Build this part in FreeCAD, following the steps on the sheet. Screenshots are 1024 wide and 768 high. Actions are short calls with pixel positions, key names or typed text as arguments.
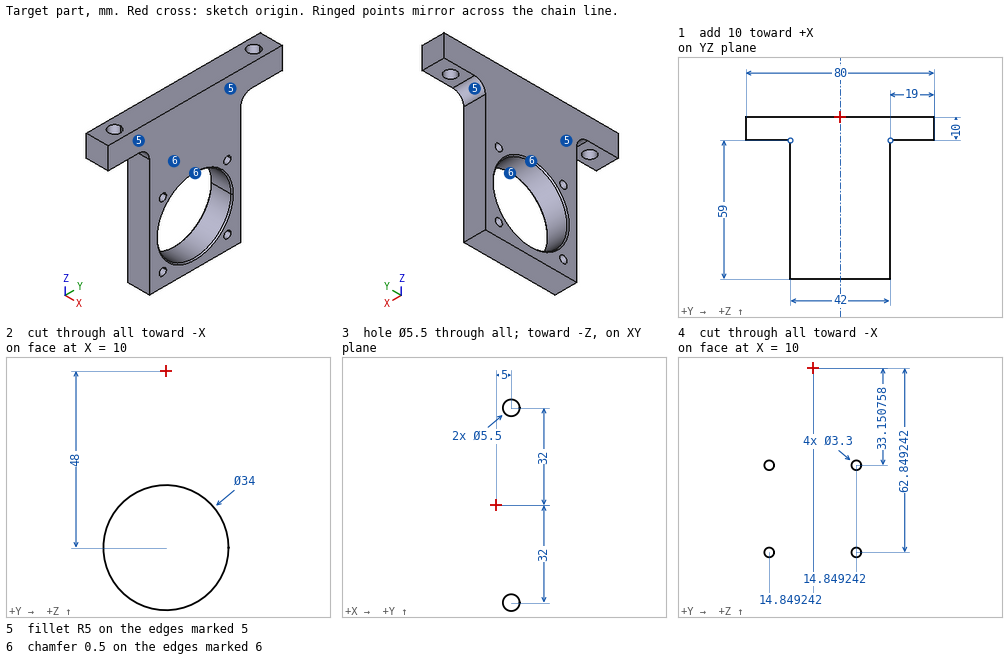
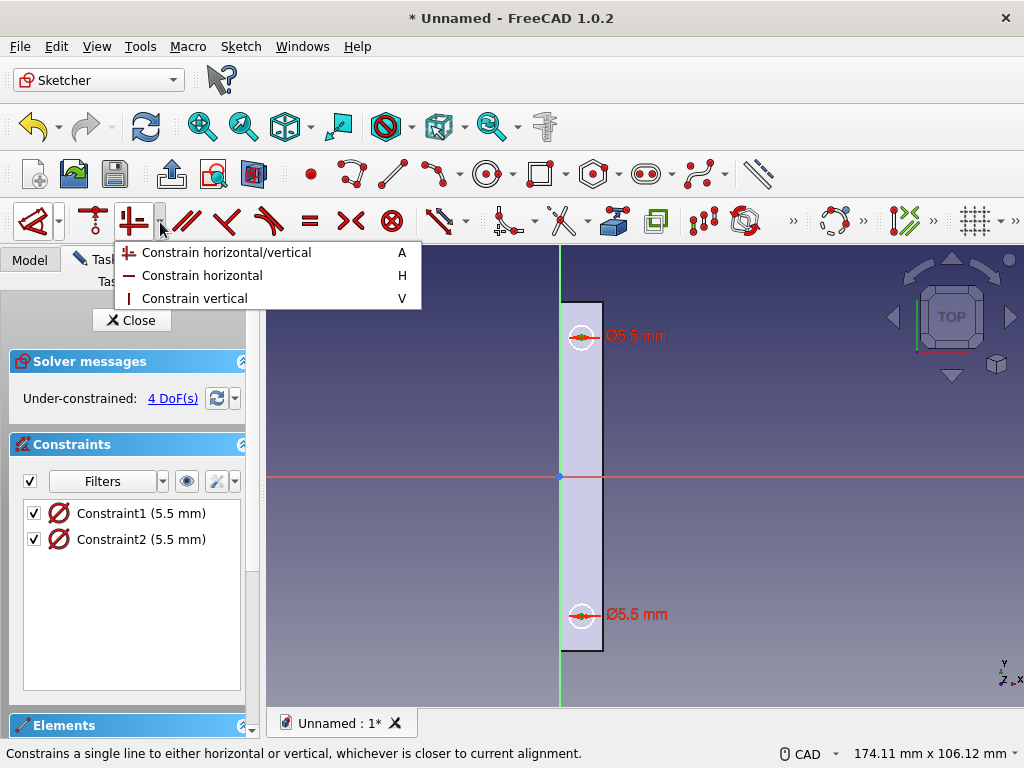
click(268, 298)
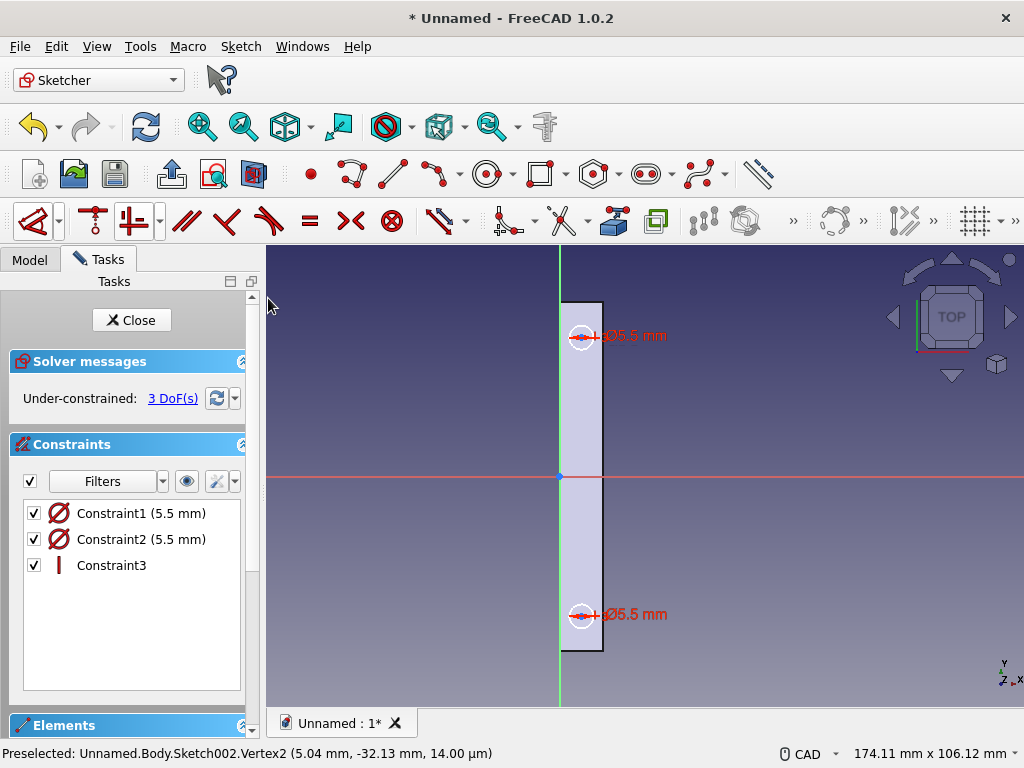
scroll(581, 338, up, 4)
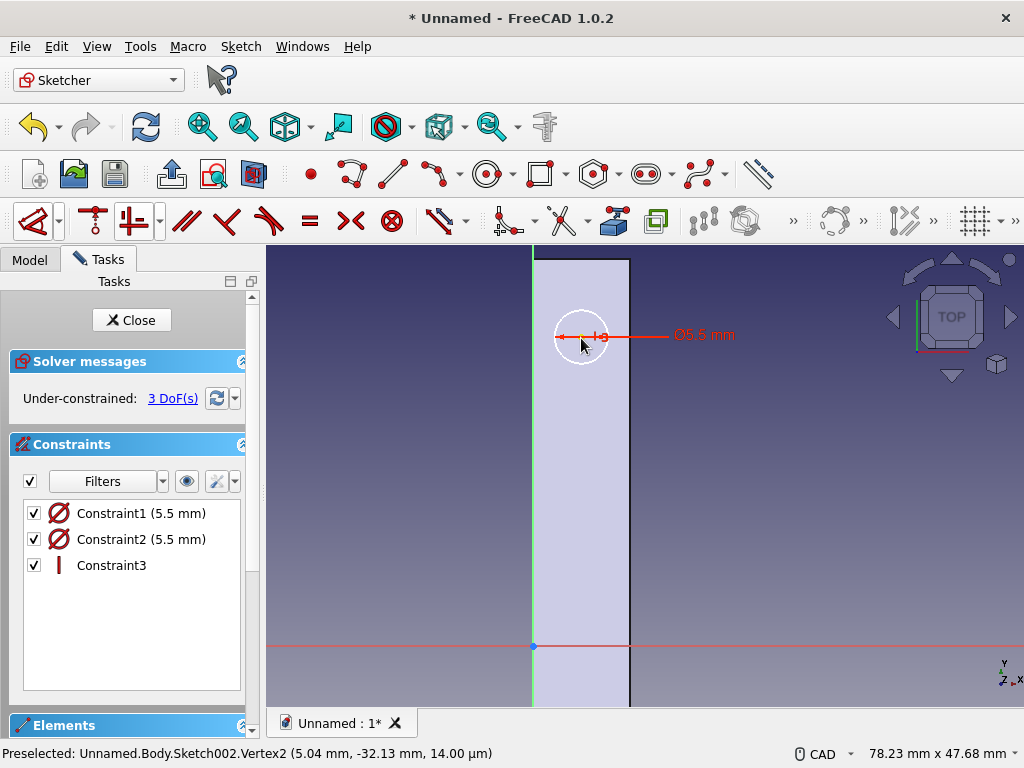
click(581, 337)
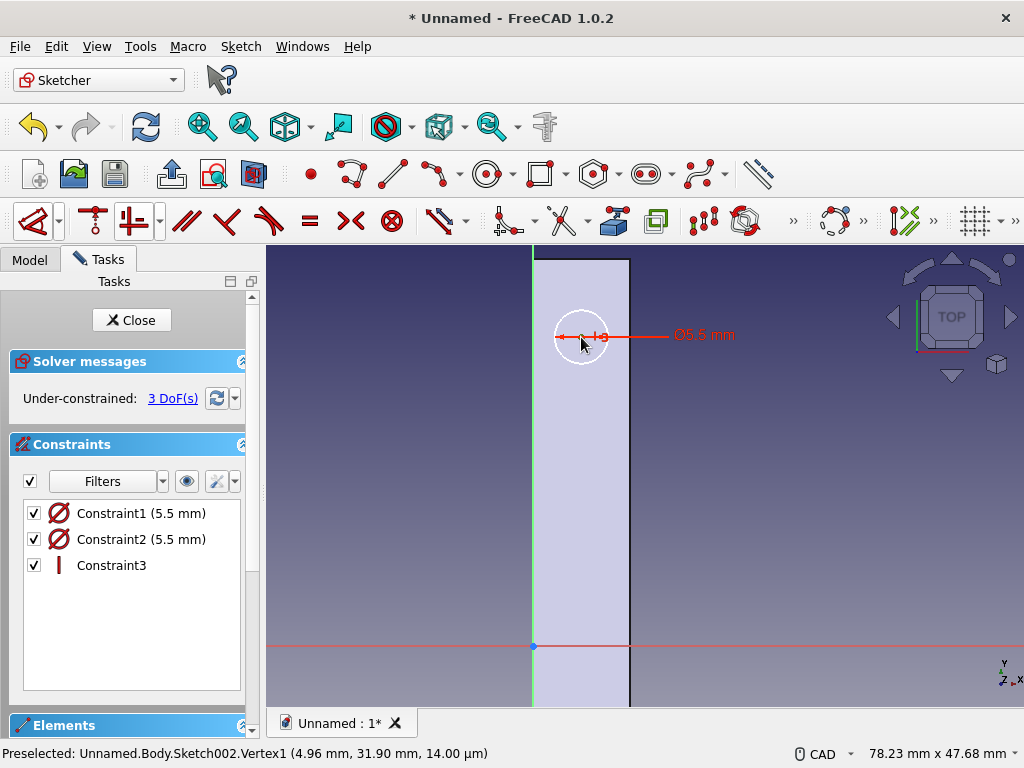
key(l)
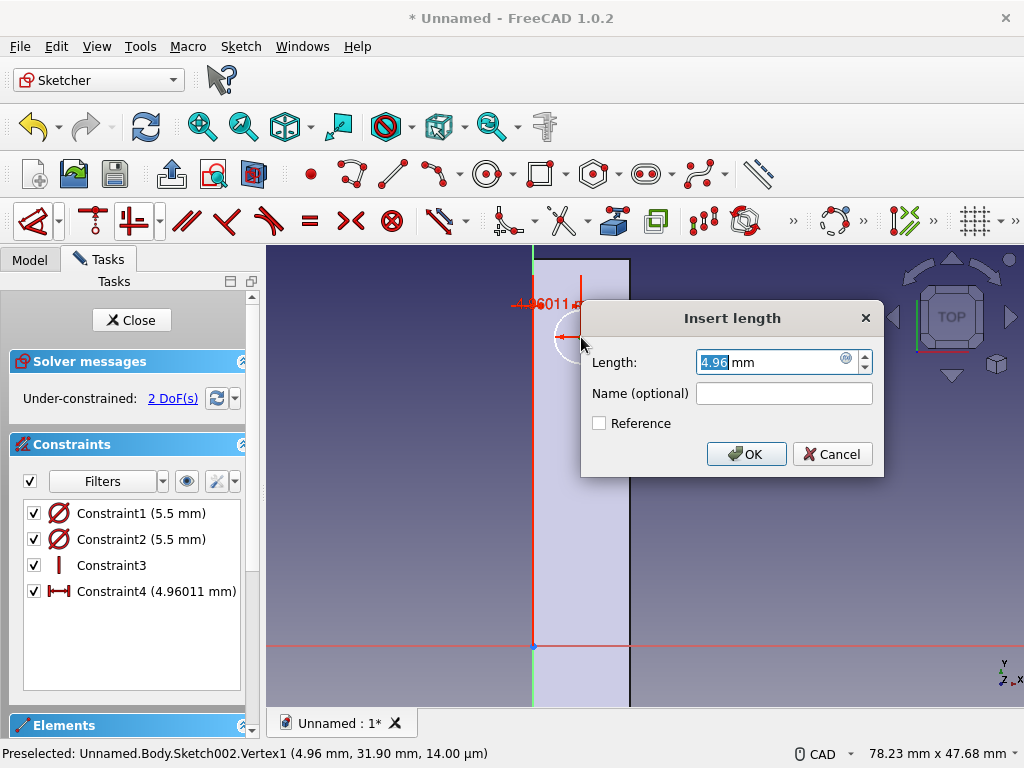
text(5)
key(Return)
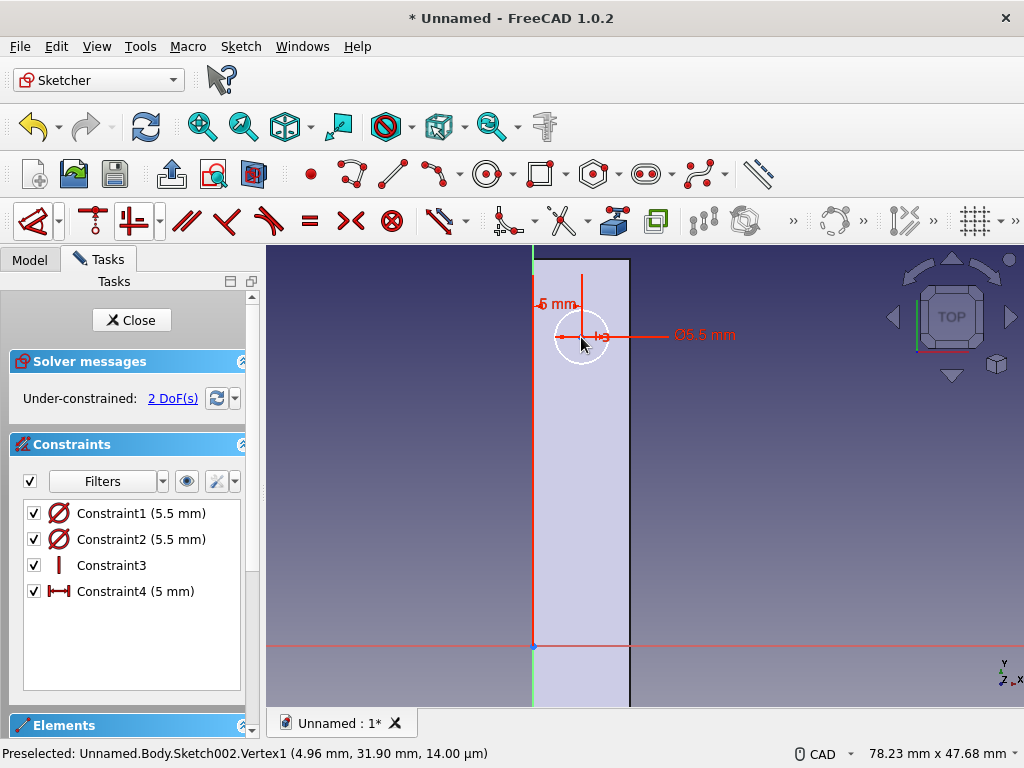
click(582, 337)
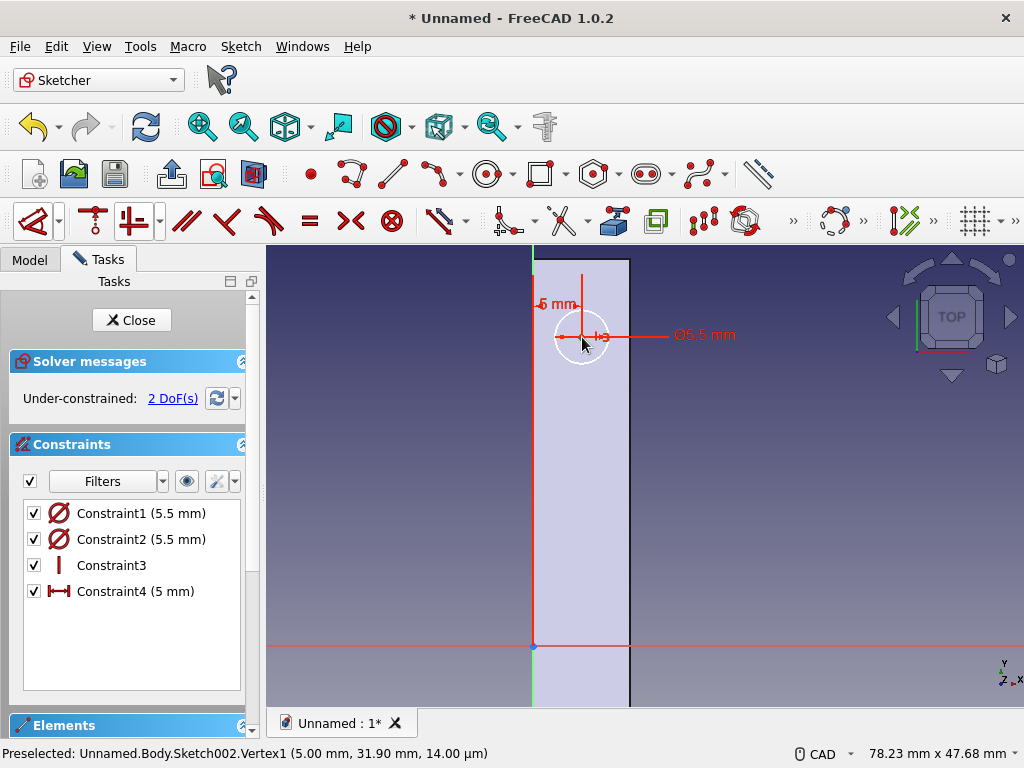
click(58, 222)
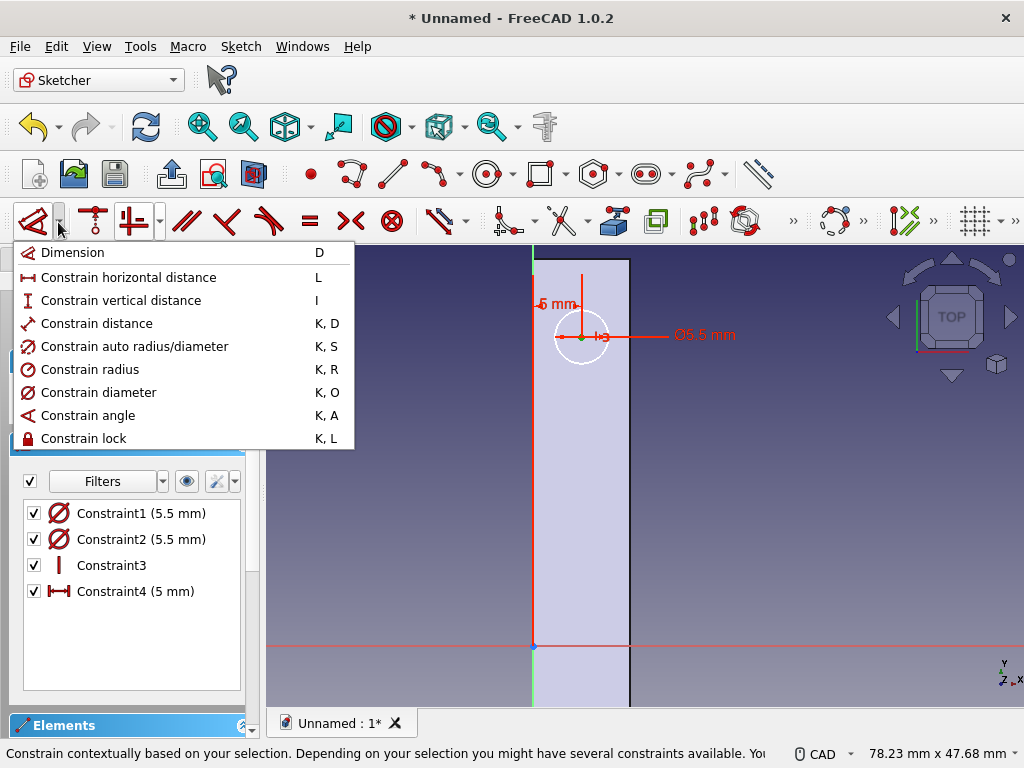
click(184, 300)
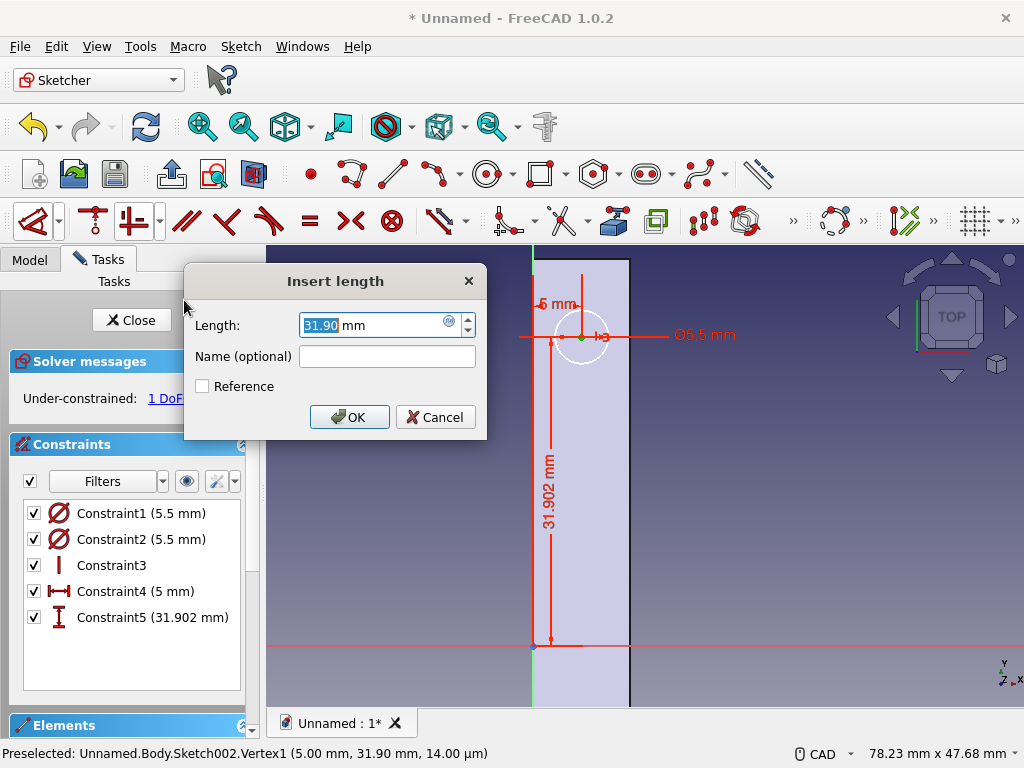
text(32)
key(Return)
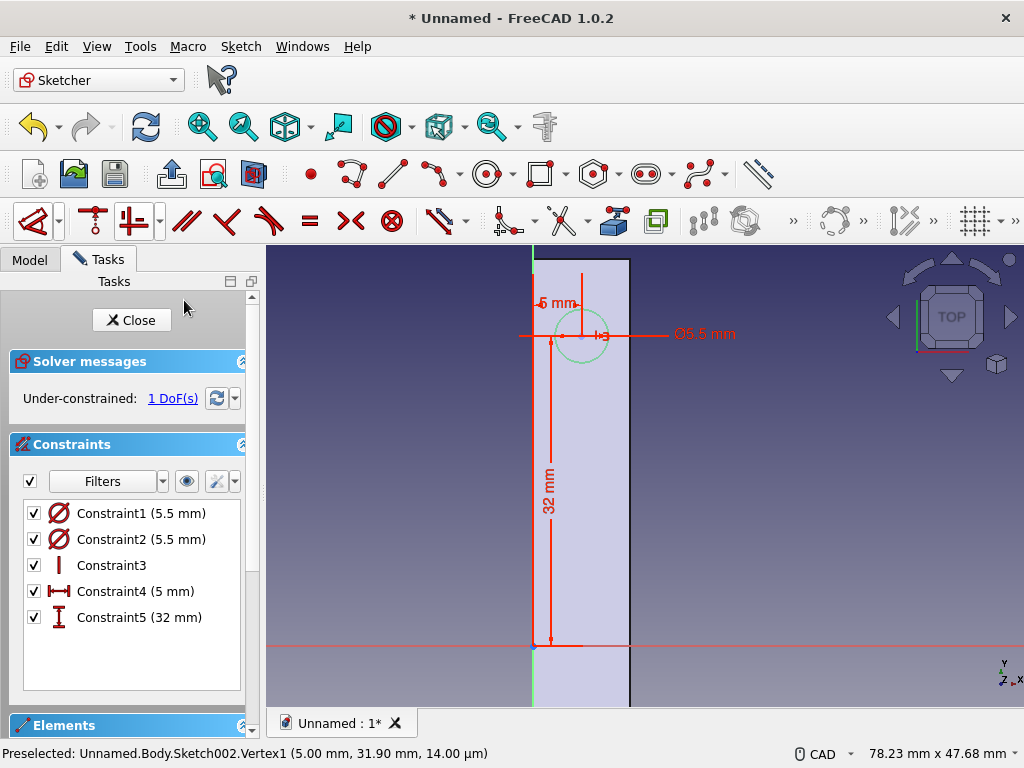
scroll(581, 337, down, 4)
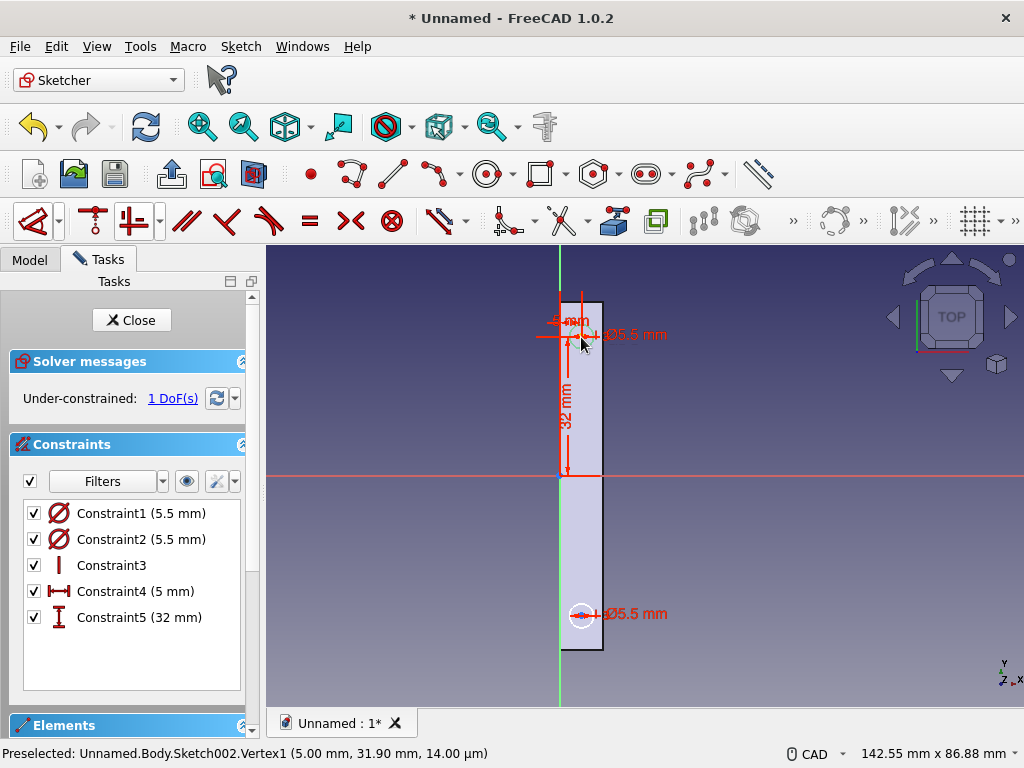
click(582, 616)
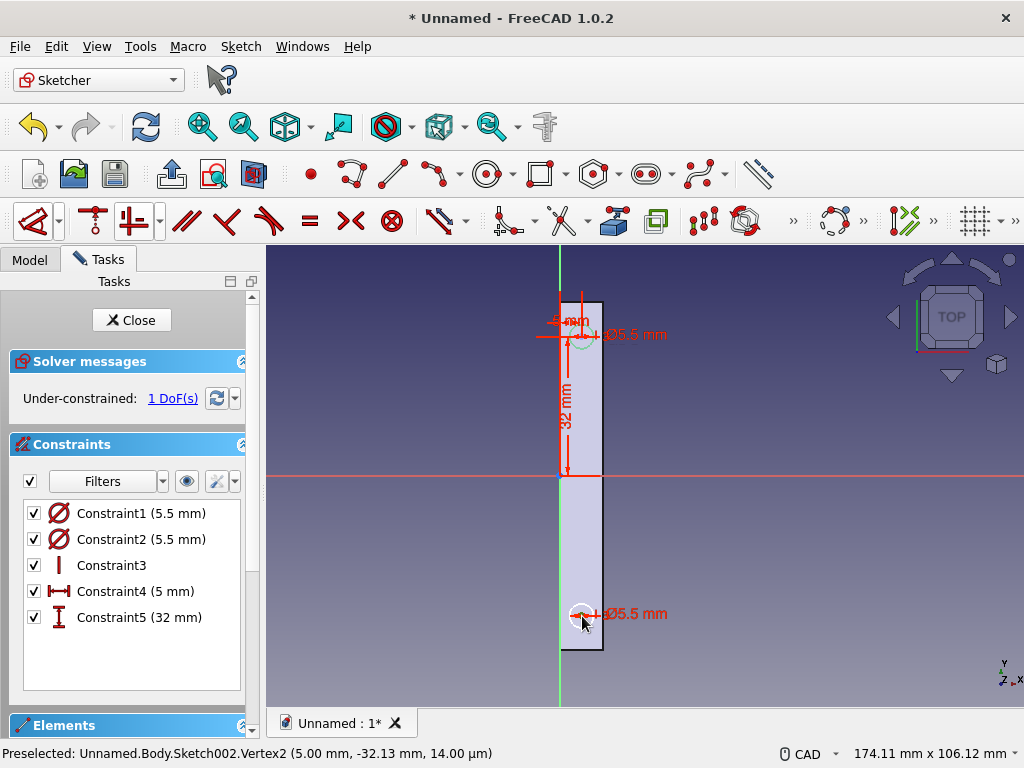
click(58, 222)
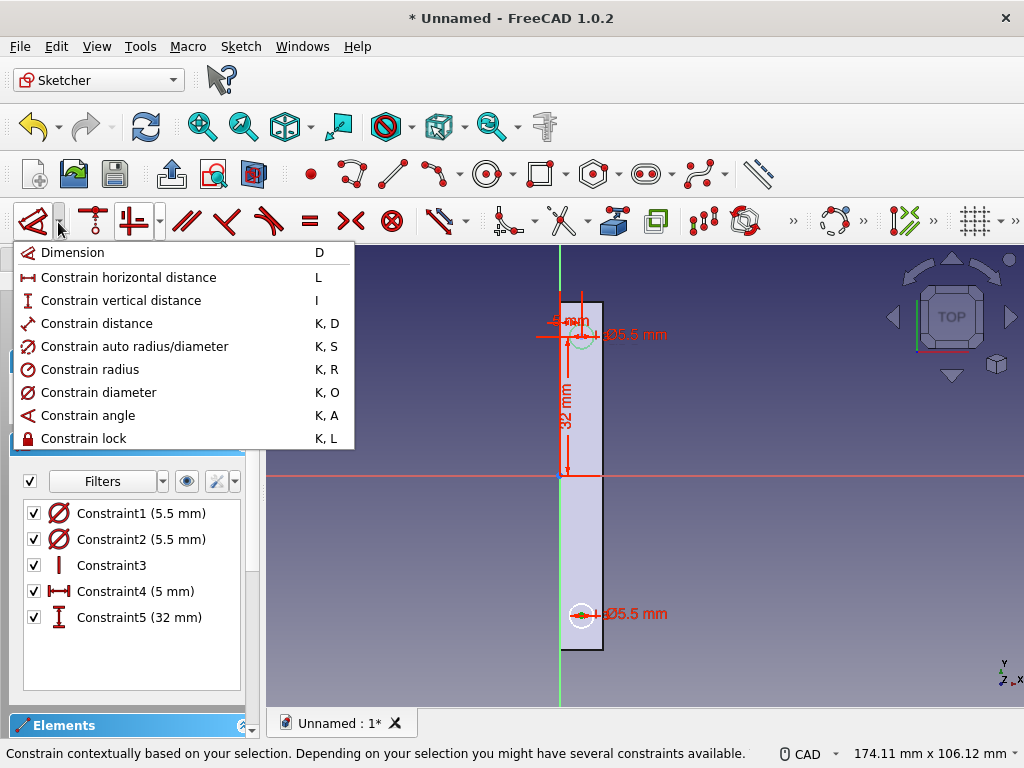
click(184, 300)